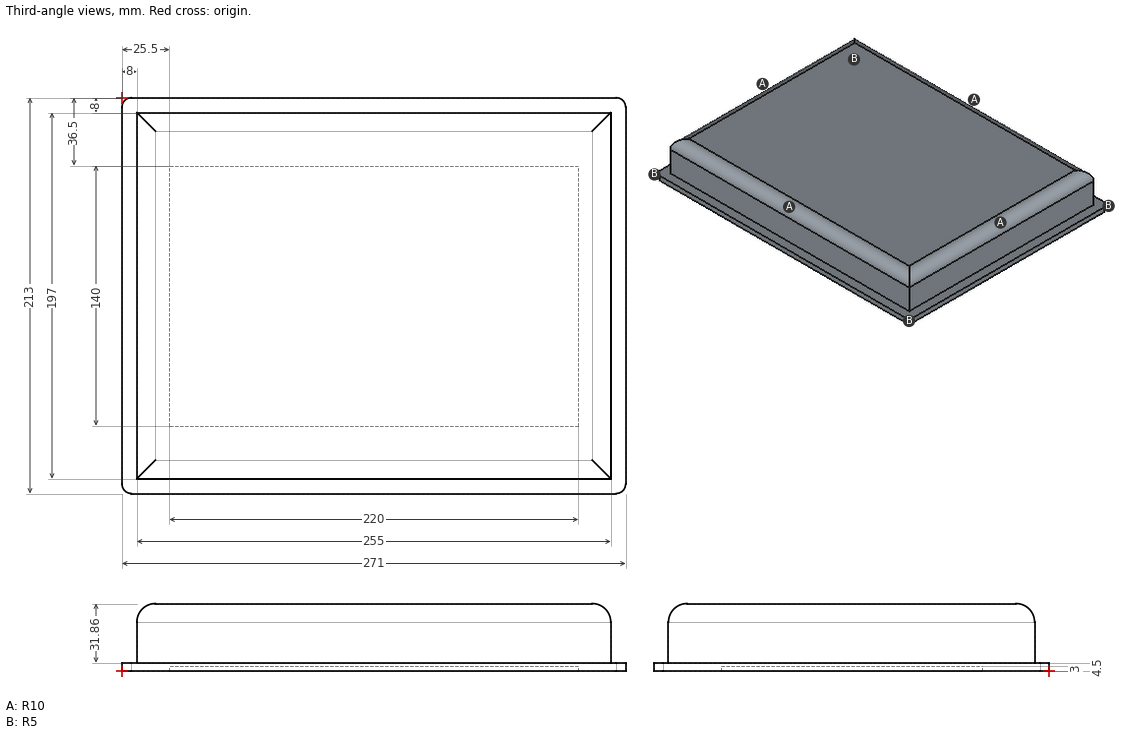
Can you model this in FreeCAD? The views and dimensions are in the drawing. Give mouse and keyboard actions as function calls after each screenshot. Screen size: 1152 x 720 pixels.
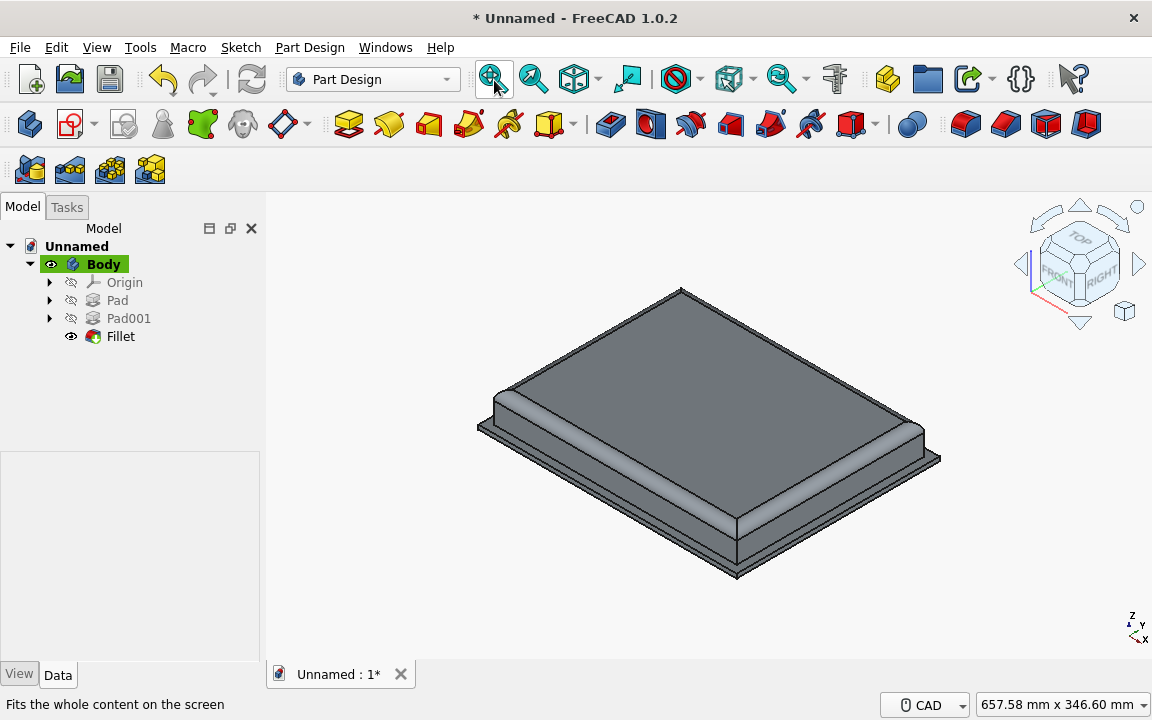
scroll(681, 309, up, 10)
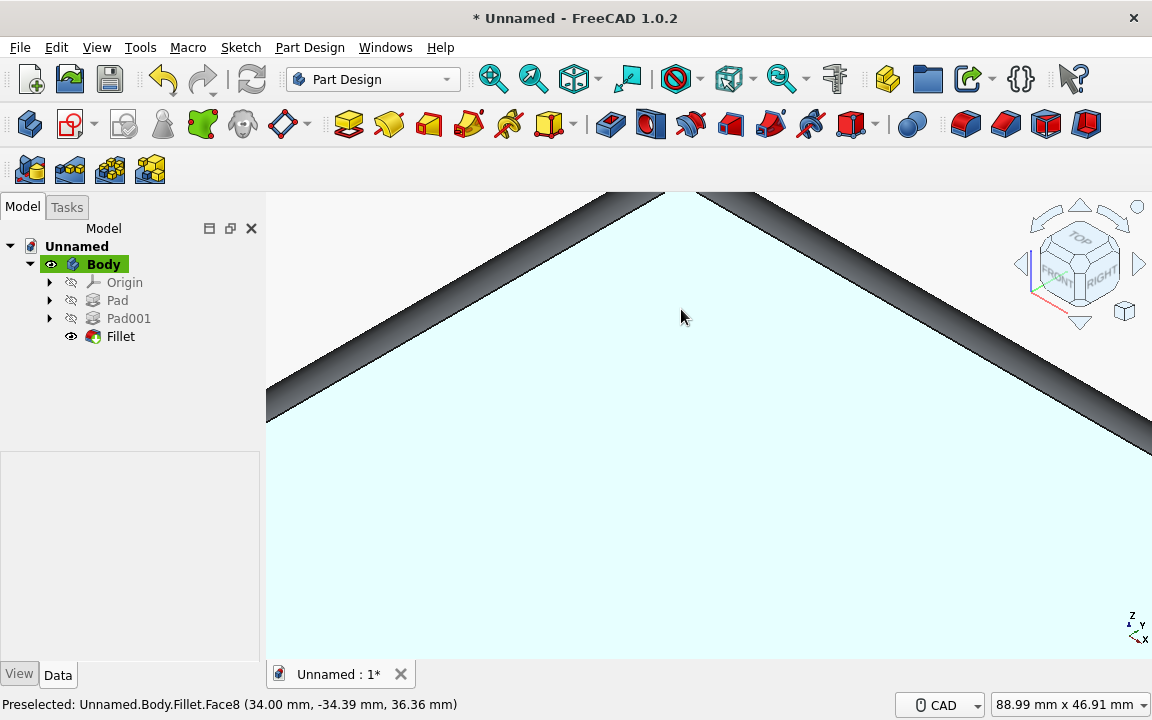
click(494, 80)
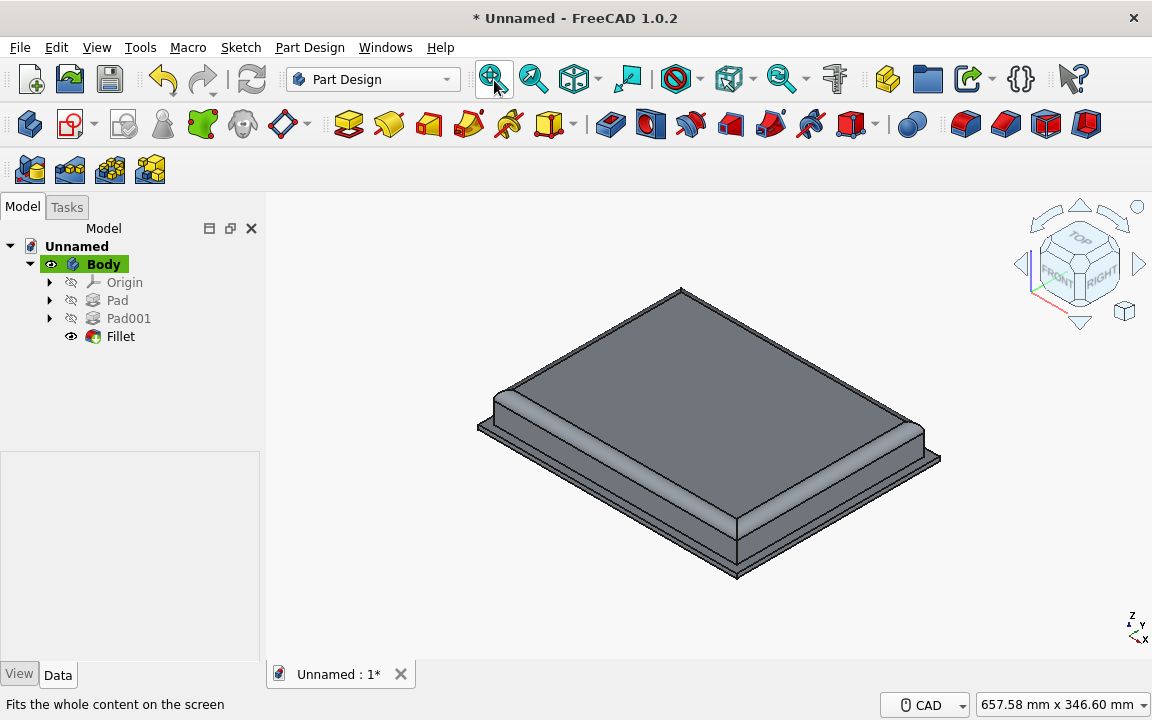
key(2)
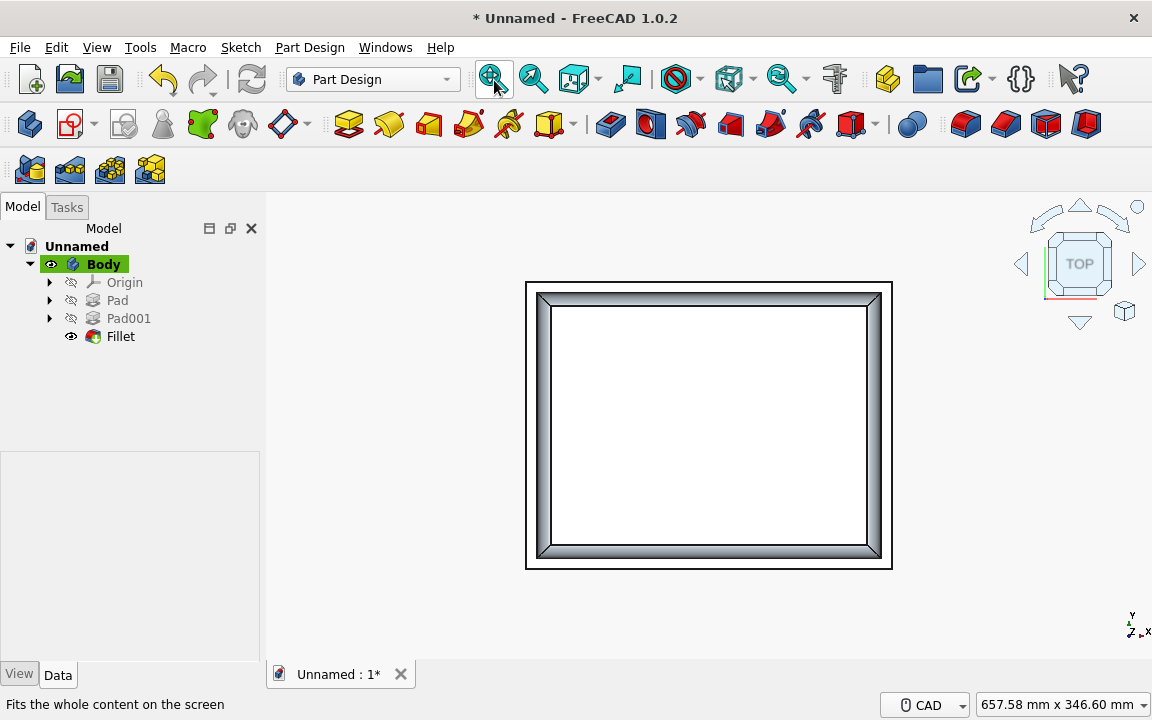
scroll(526, 281, up, 10)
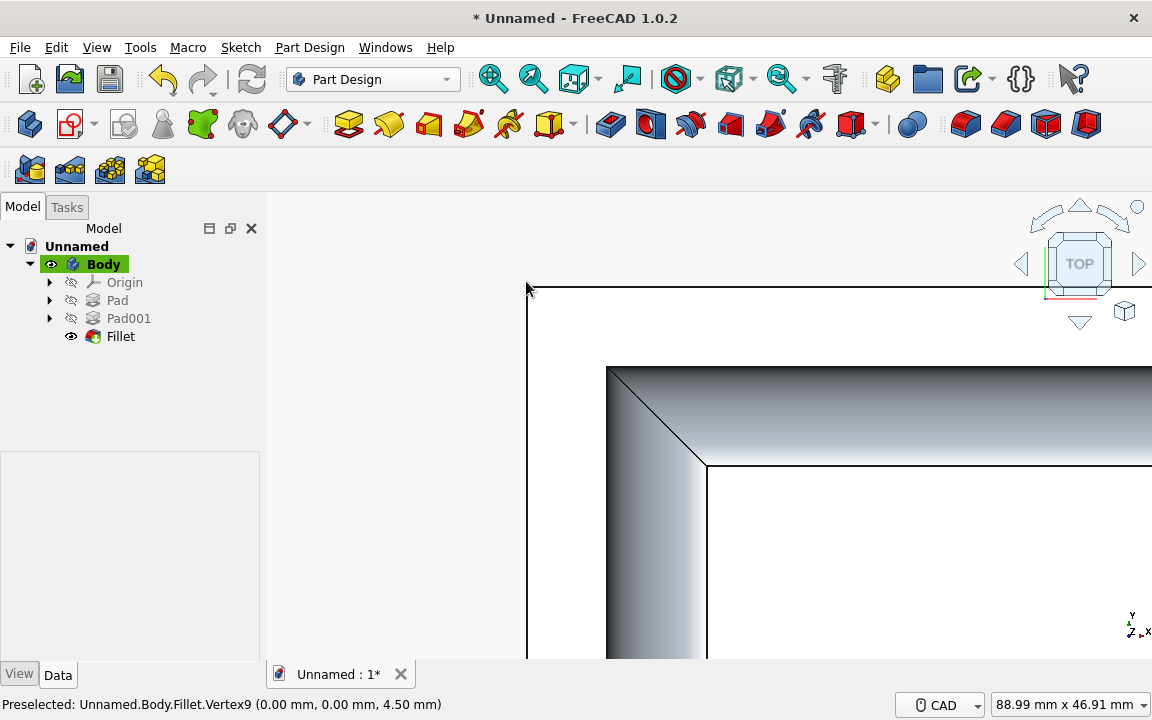
click(494, 80)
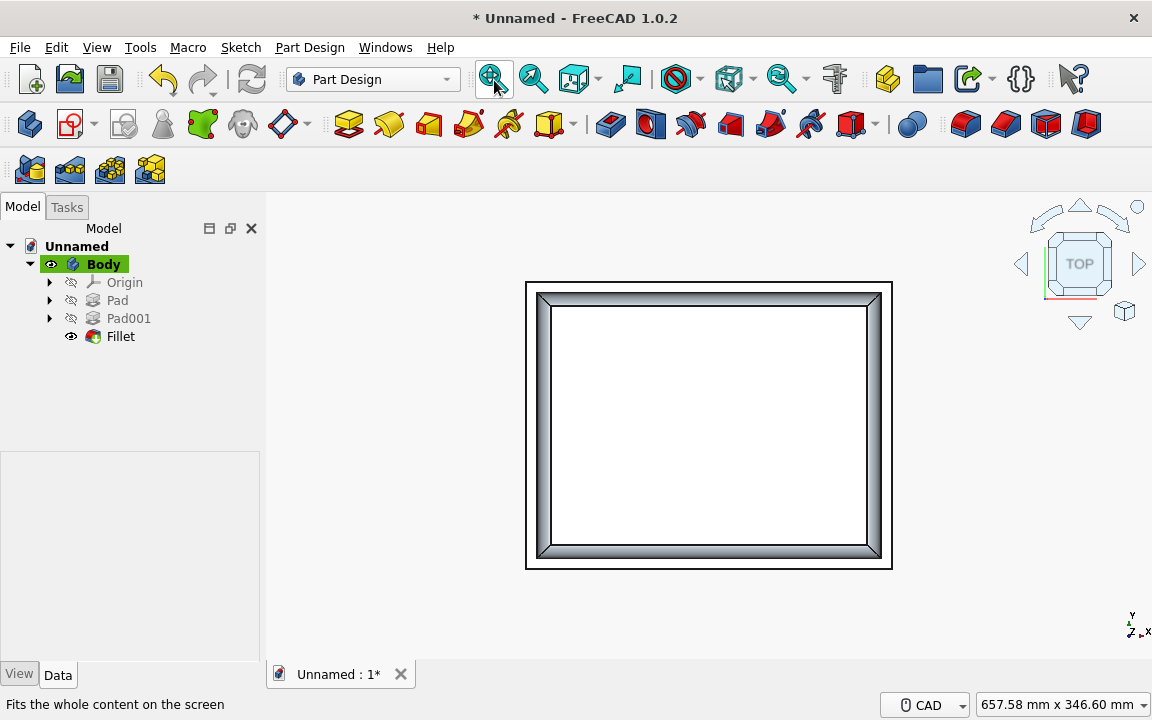
key(1)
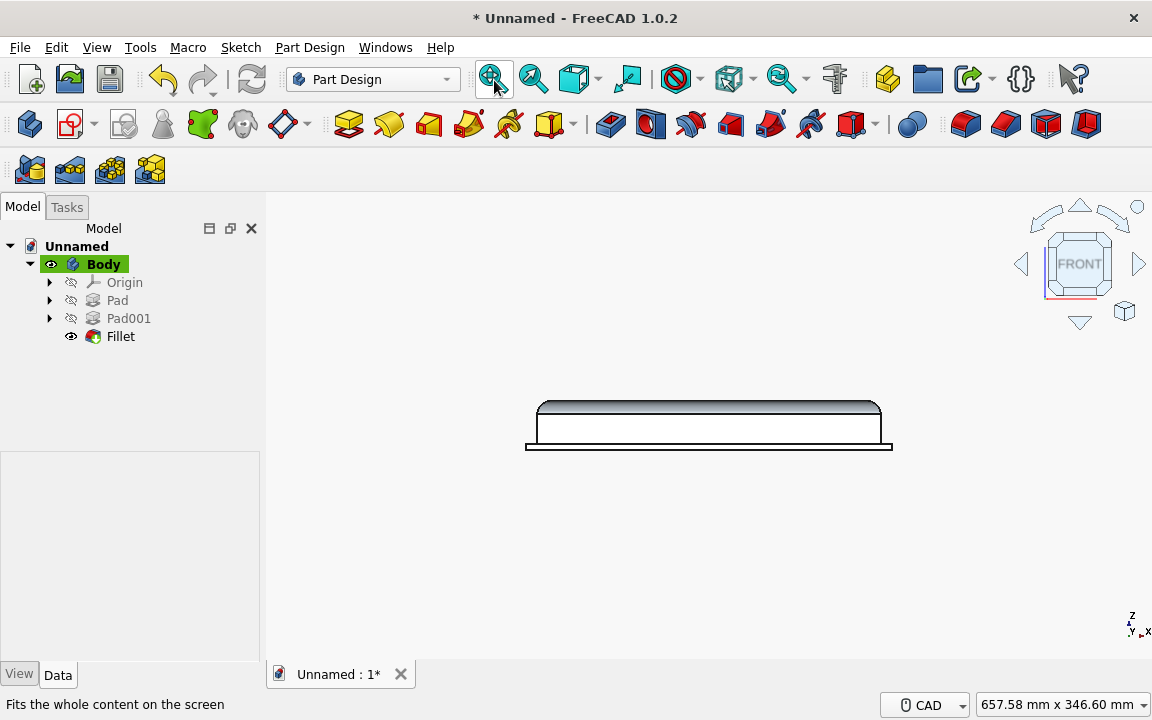
click(494, 80)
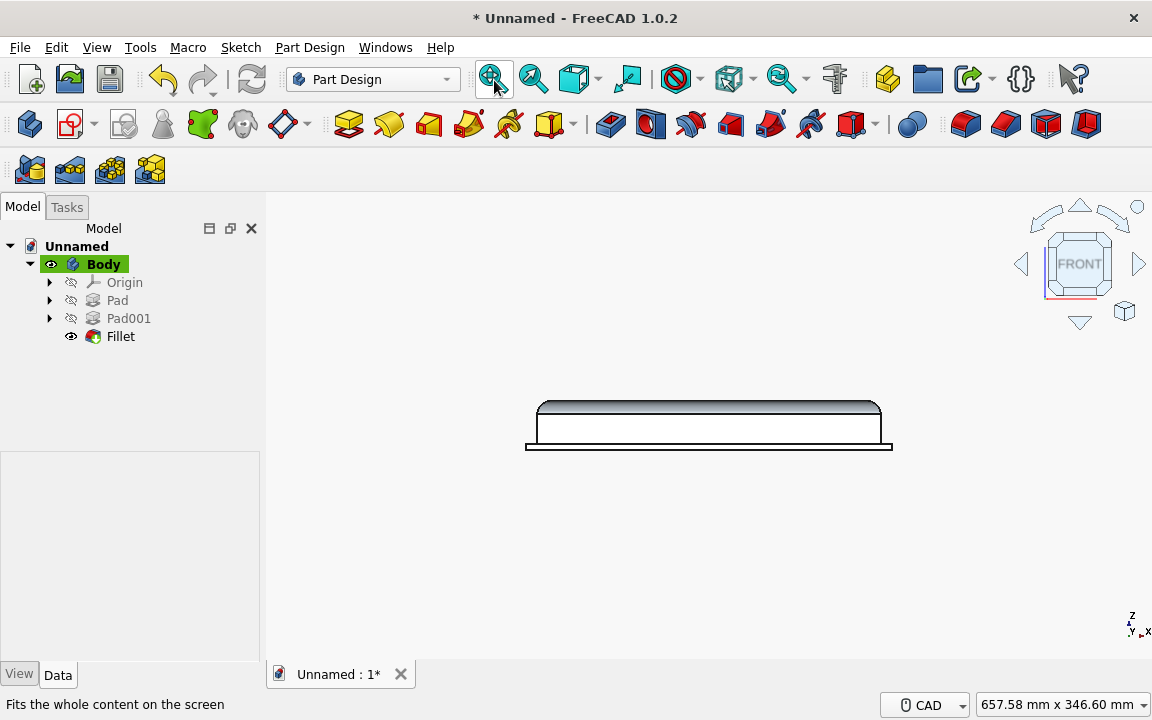
scroll(526, 446, up, 10)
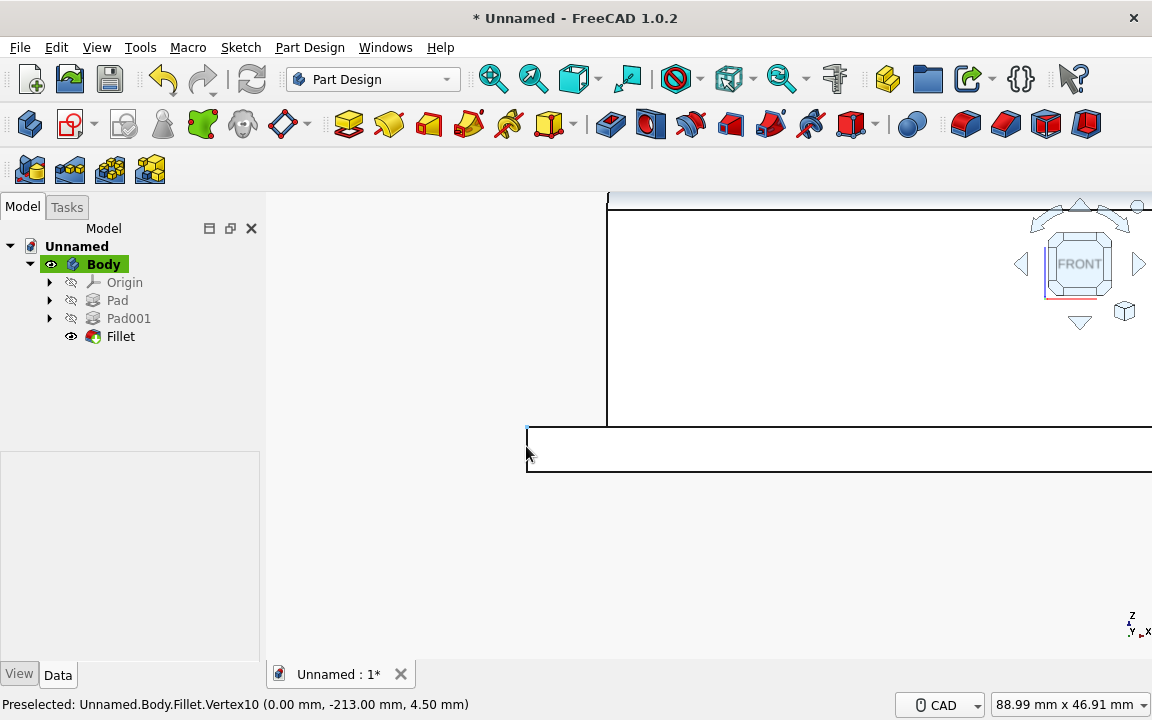
click(527, 449)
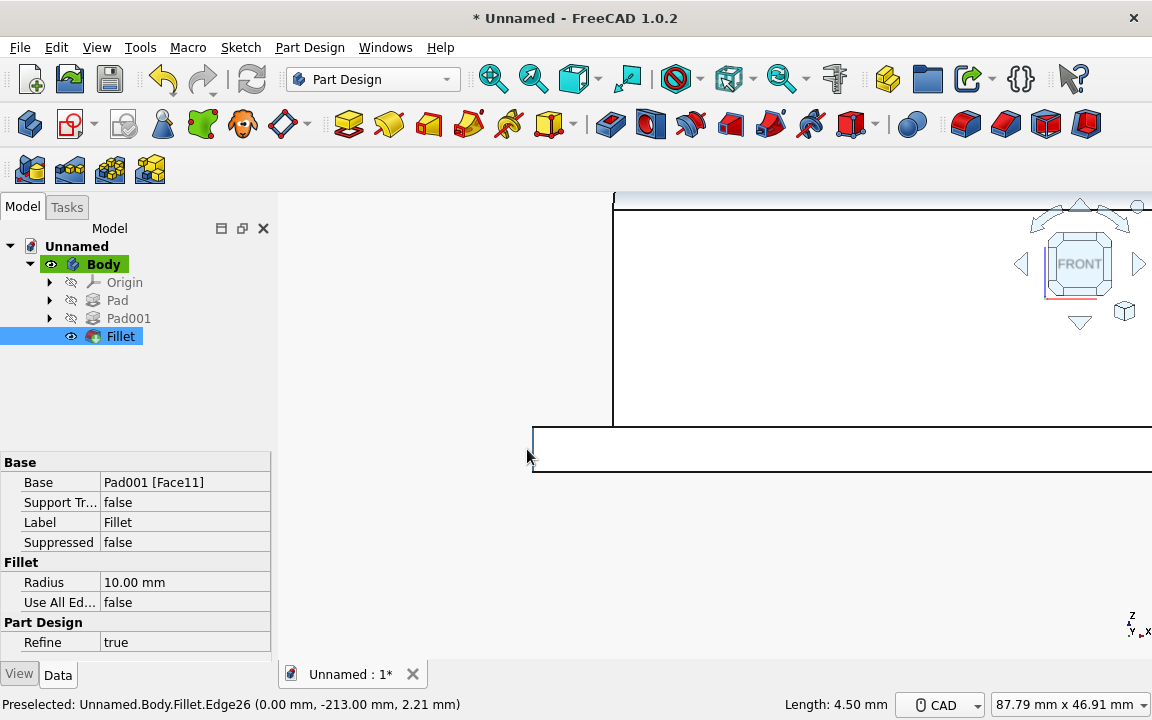
click(494, 80)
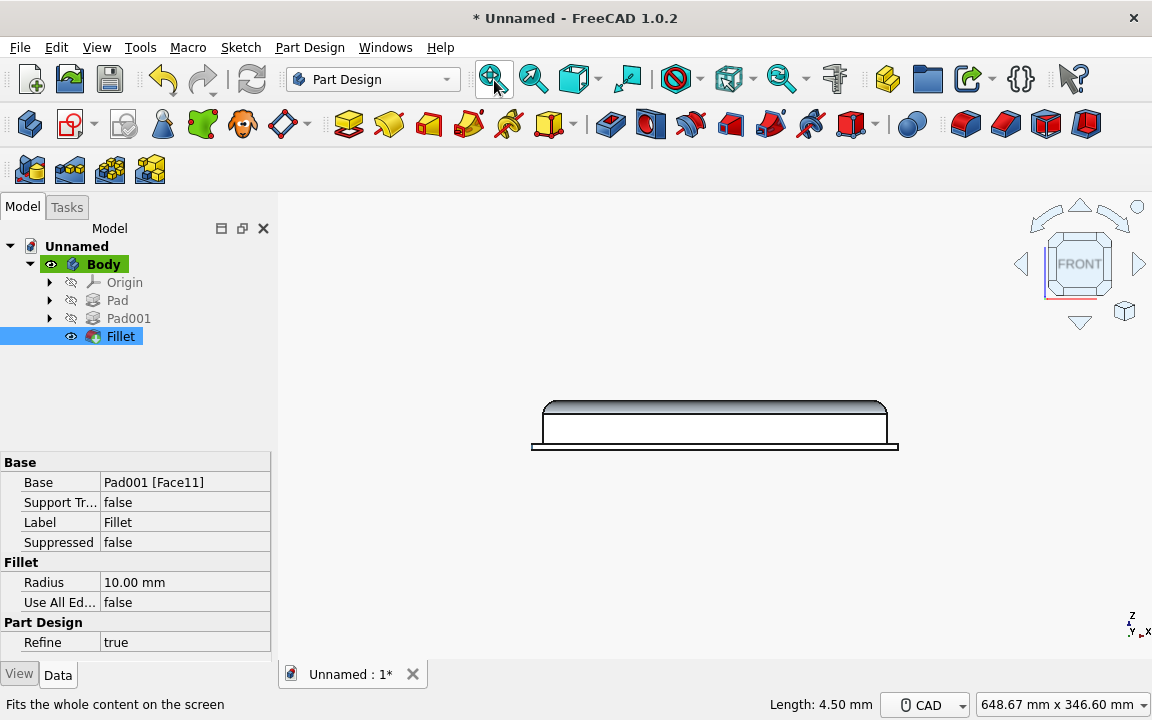
key(3)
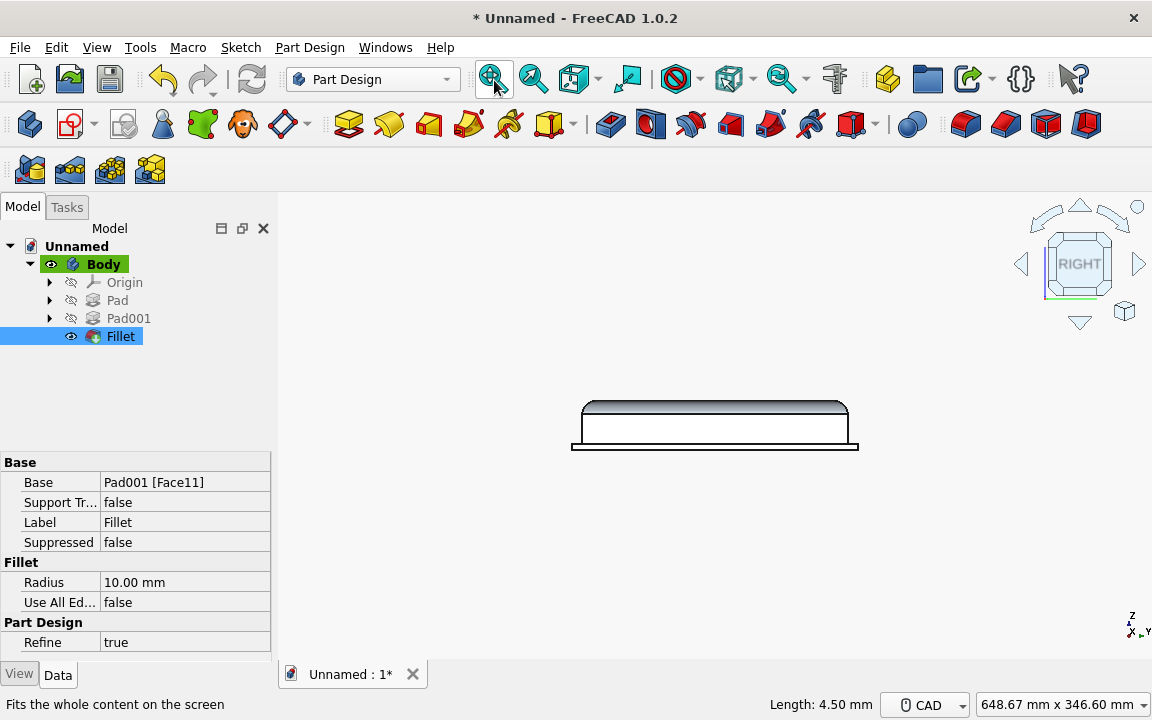
click(494, 80)